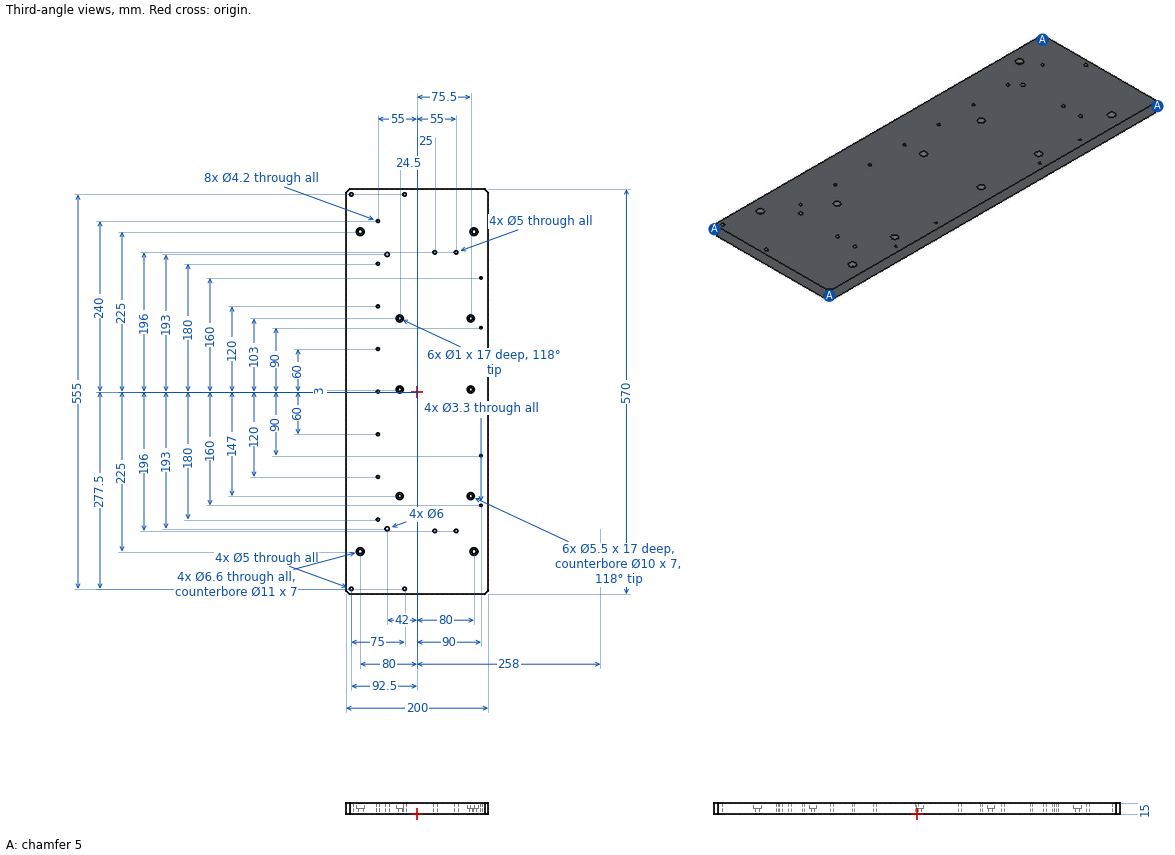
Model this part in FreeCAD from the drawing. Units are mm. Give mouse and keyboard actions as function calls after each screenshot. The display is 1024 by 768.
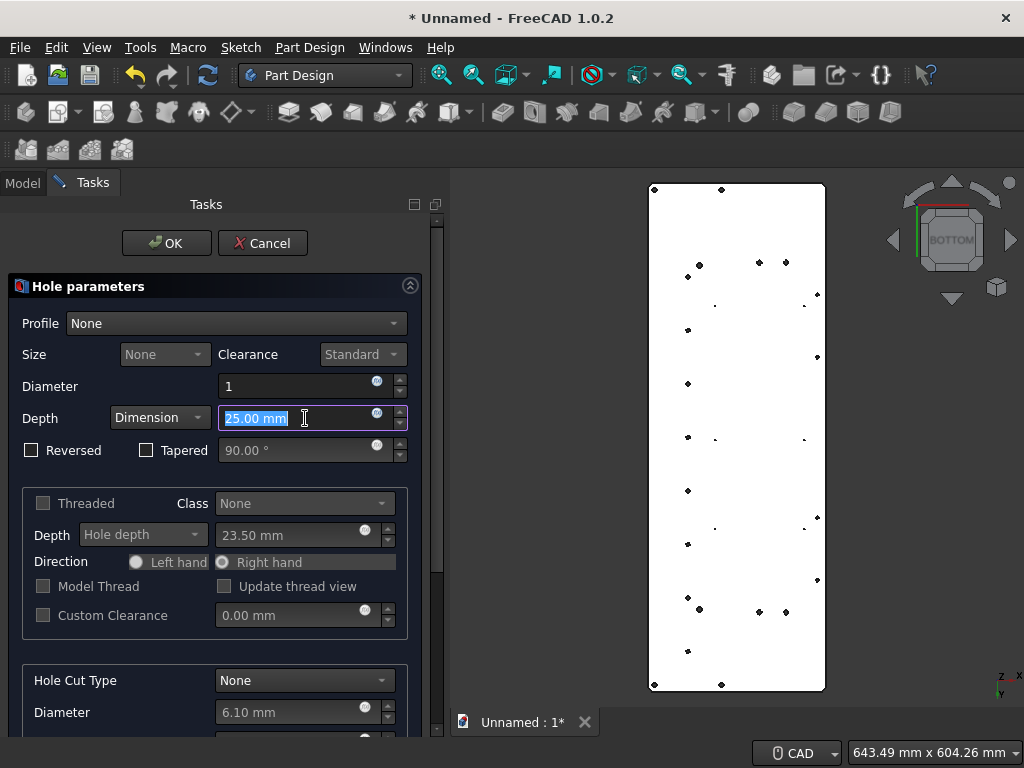
text(17)
key(Tab)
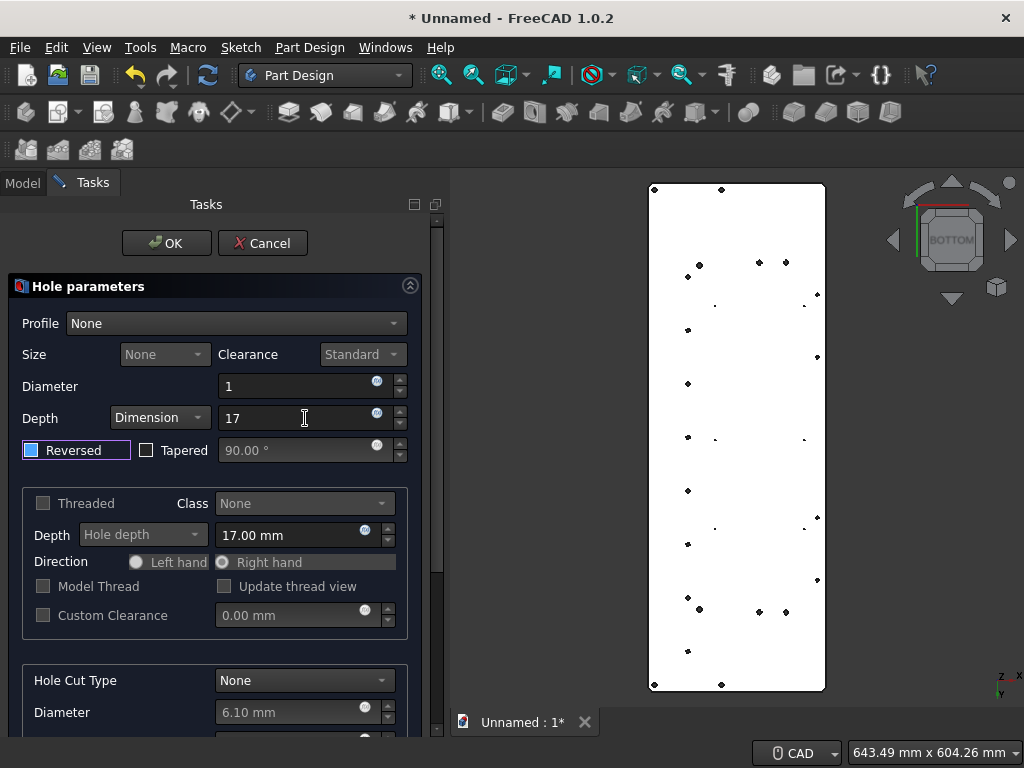
click(167, 243)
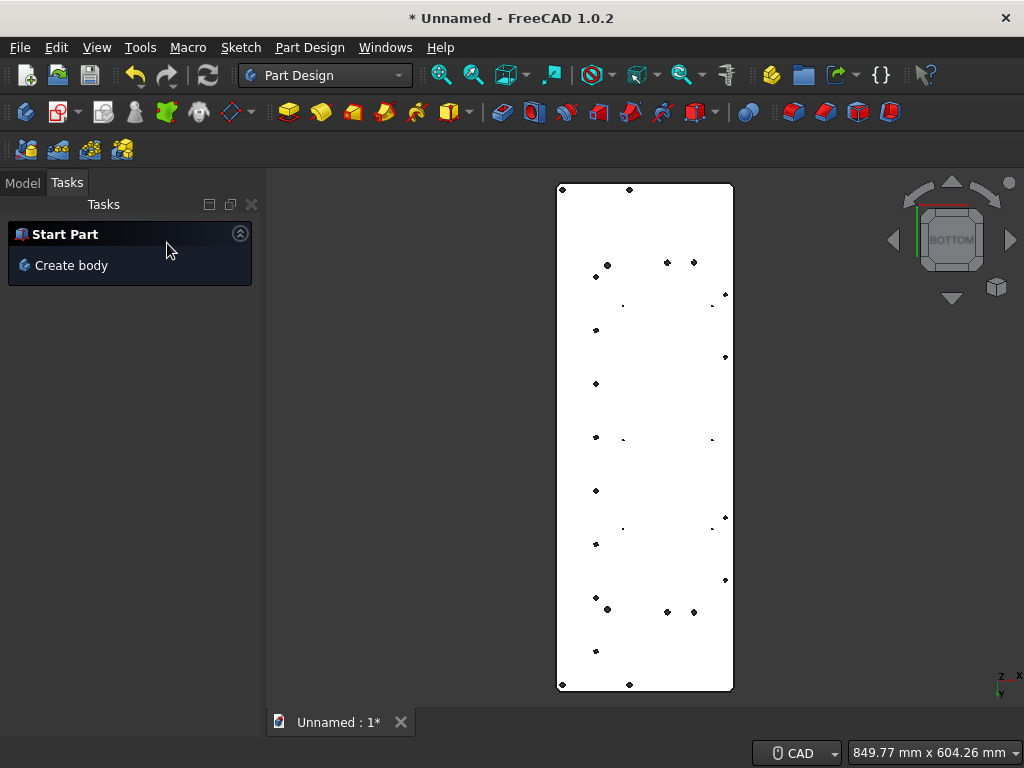
key(0)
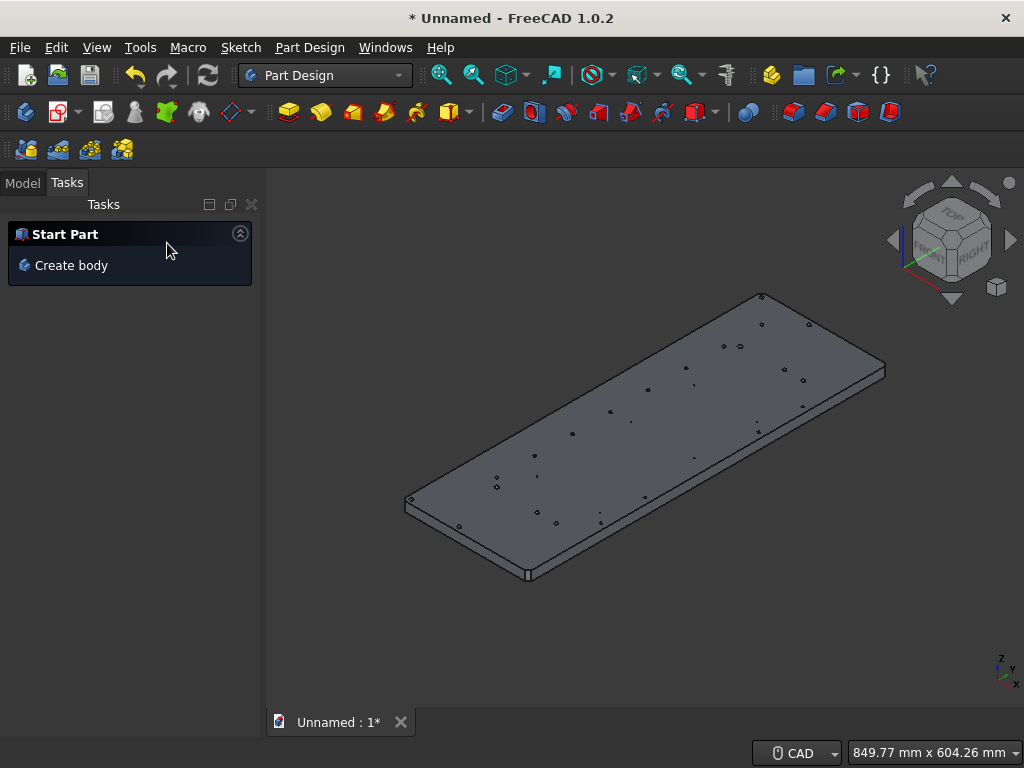
click(612, 471)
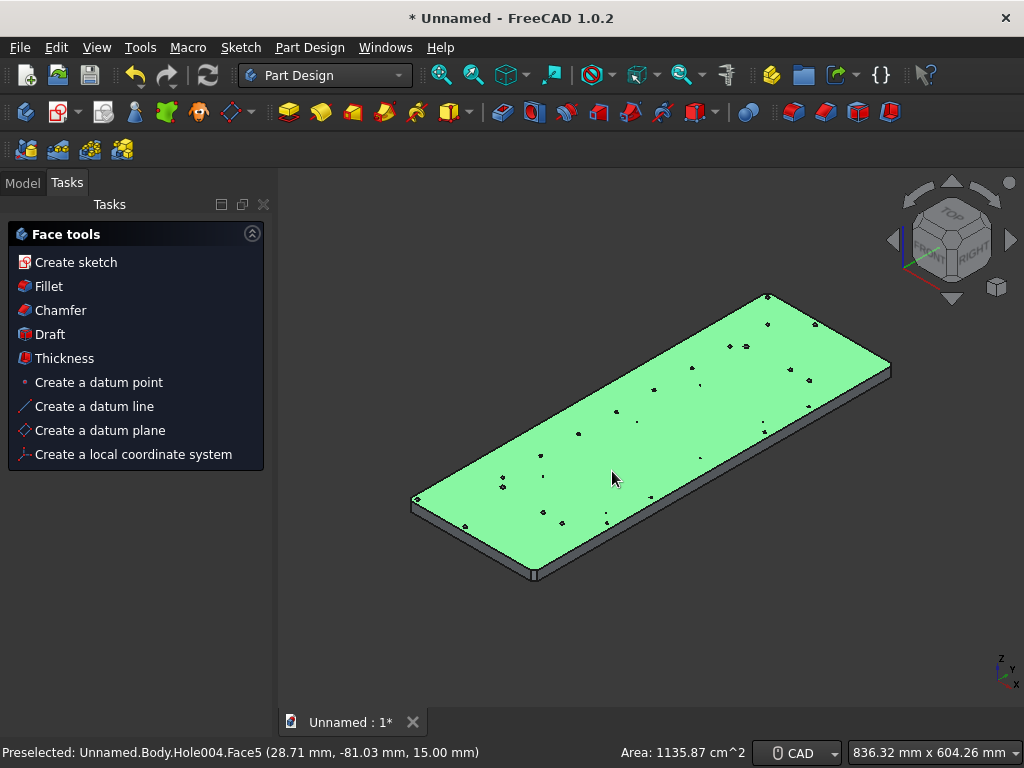
click(58, 112)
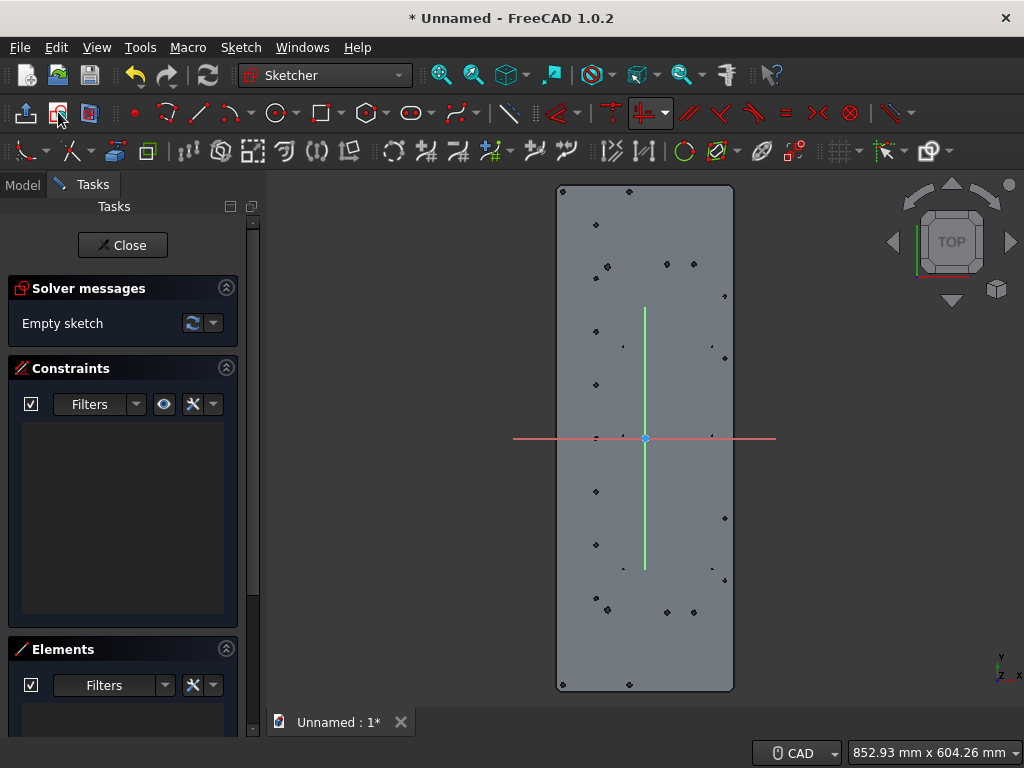
scroll(853, 498, up, 2)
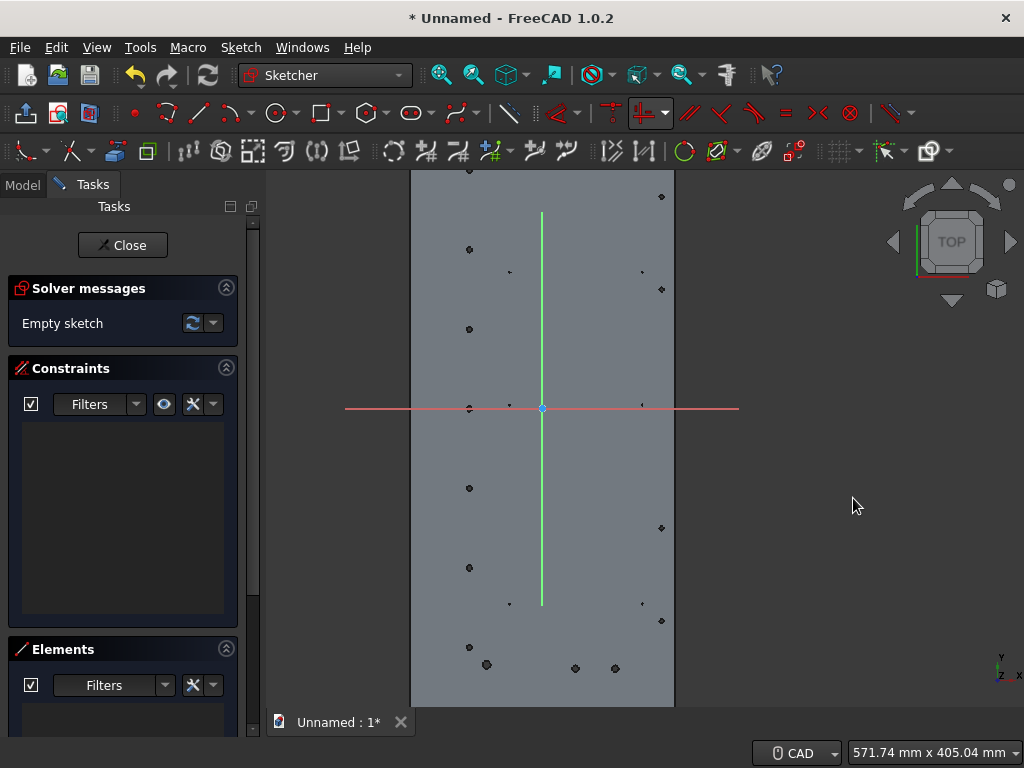
click(276, 114)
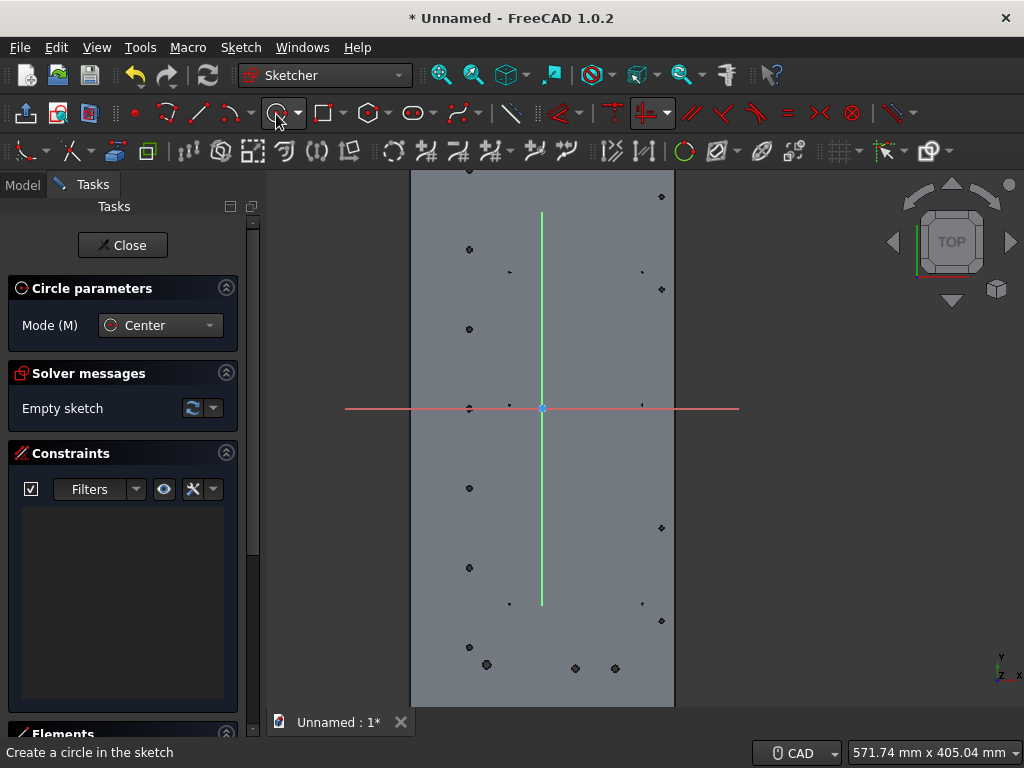
scroll(642, 604, up, 10)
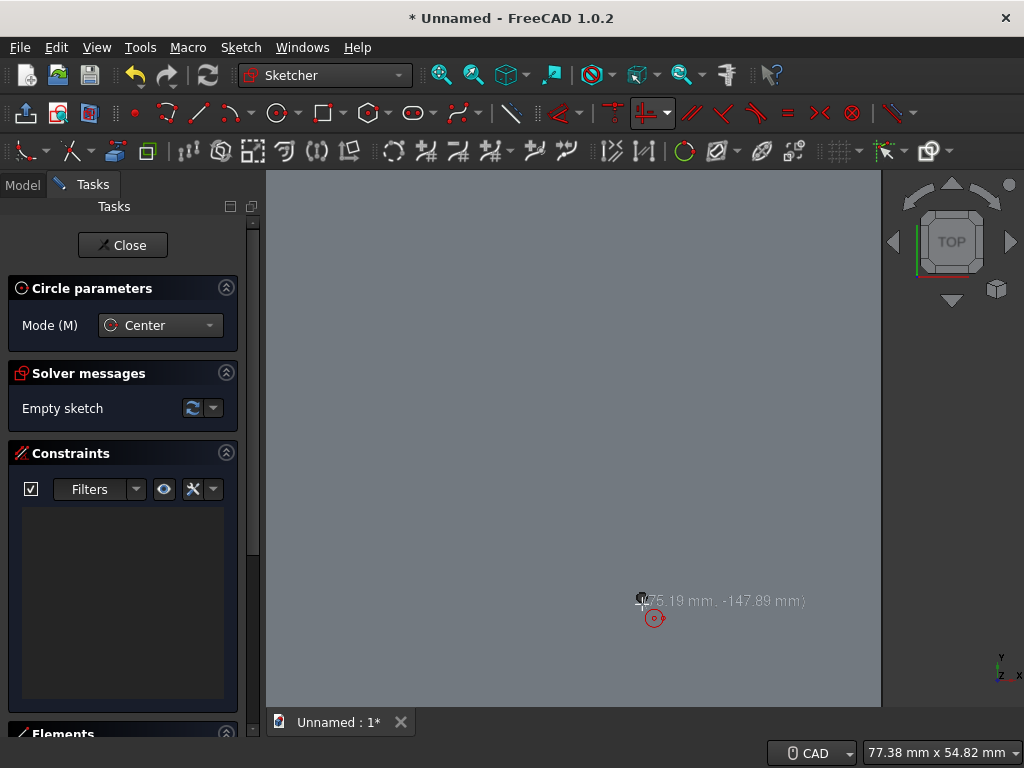
scroll(643, 605, down, 10)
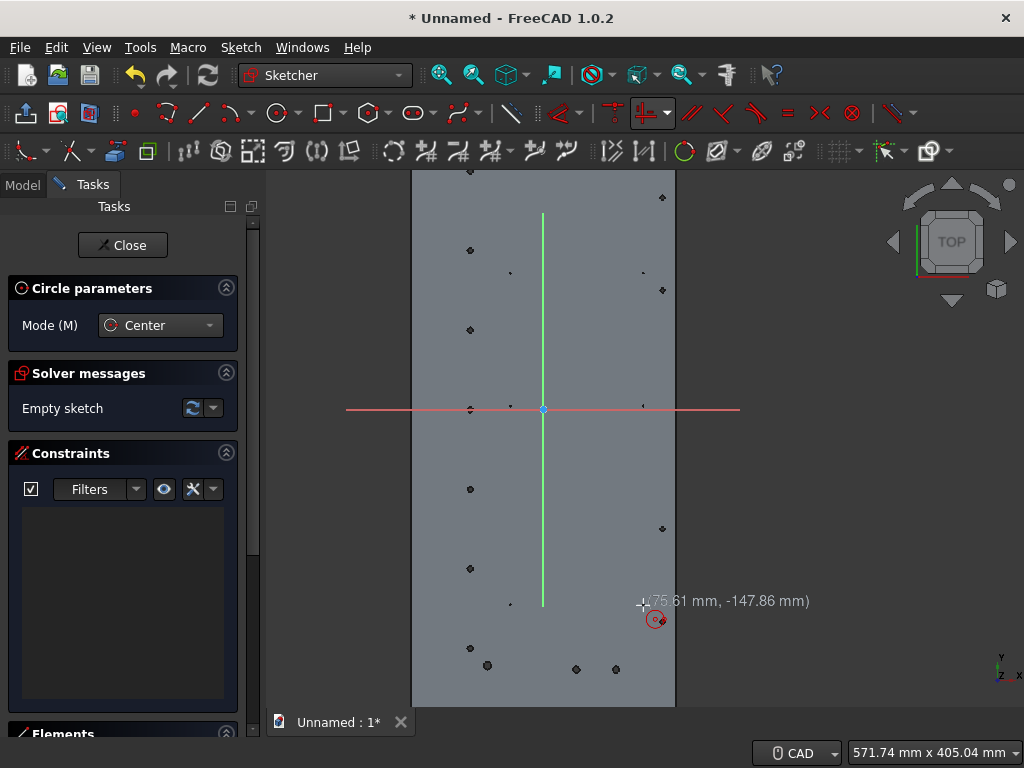
click(643, 605)
move(646, 602)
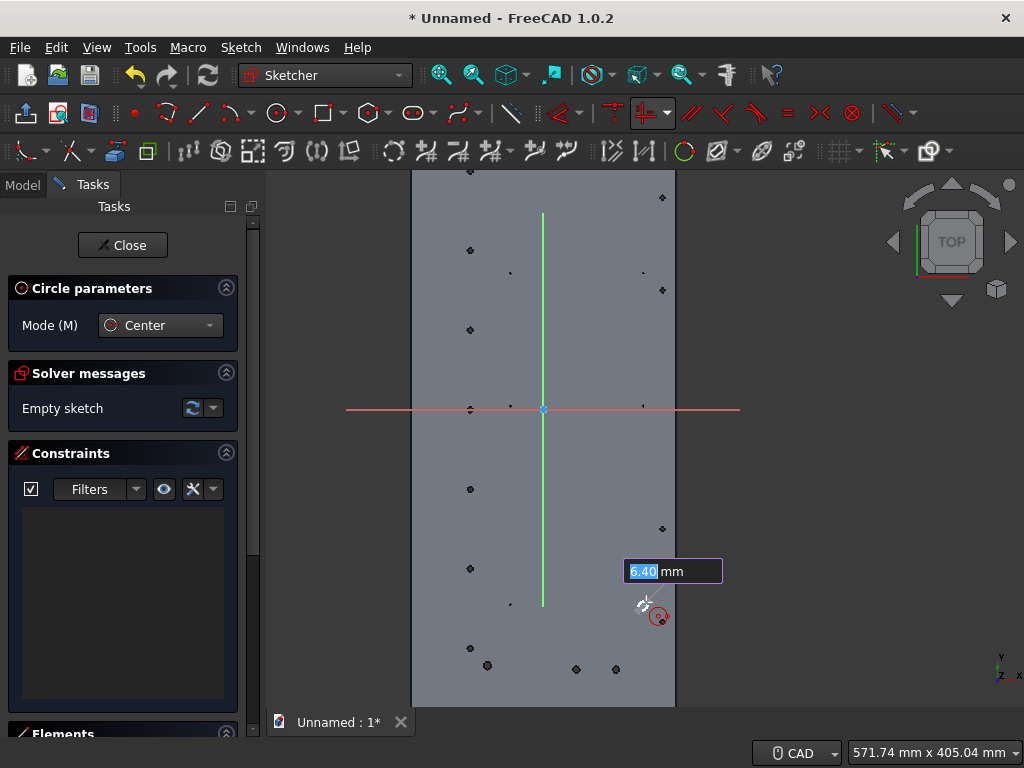
text(5.5)
key(Return)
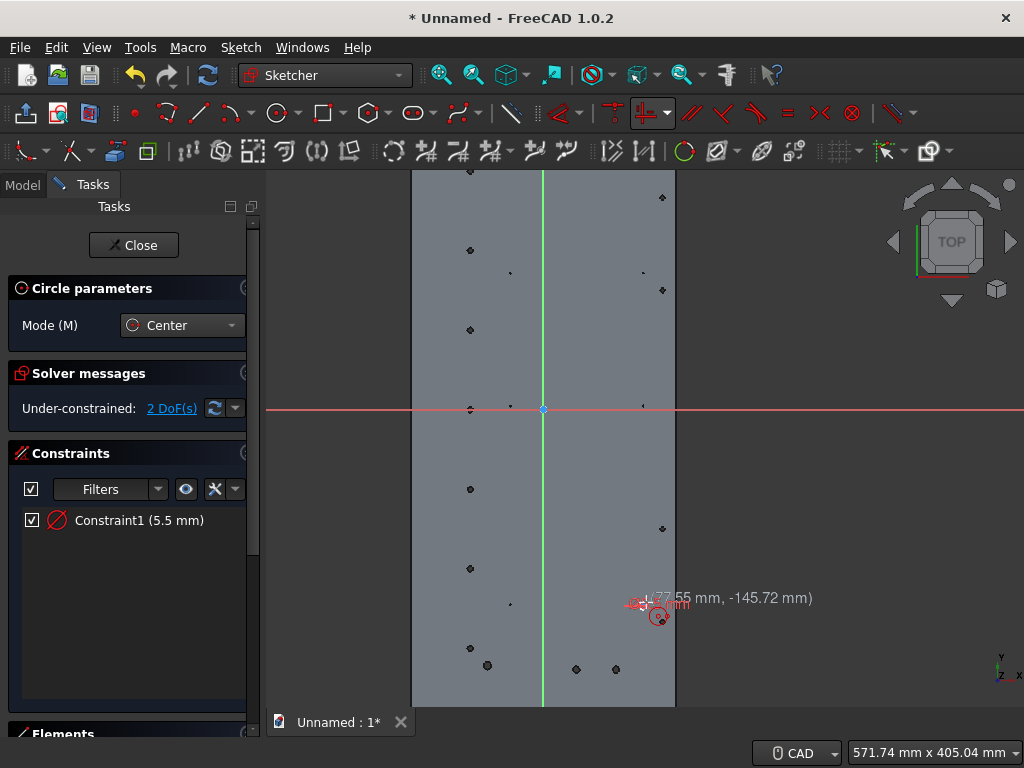
scroll(643, 273, up, 10)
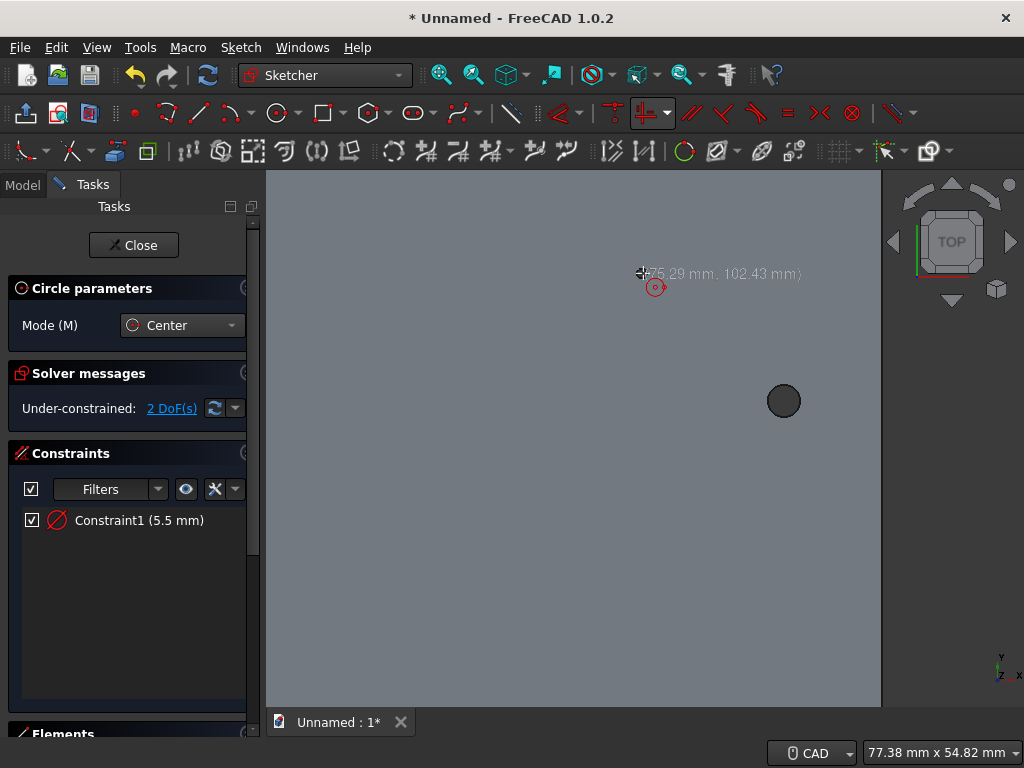
scroll(643, 273, down, 10)